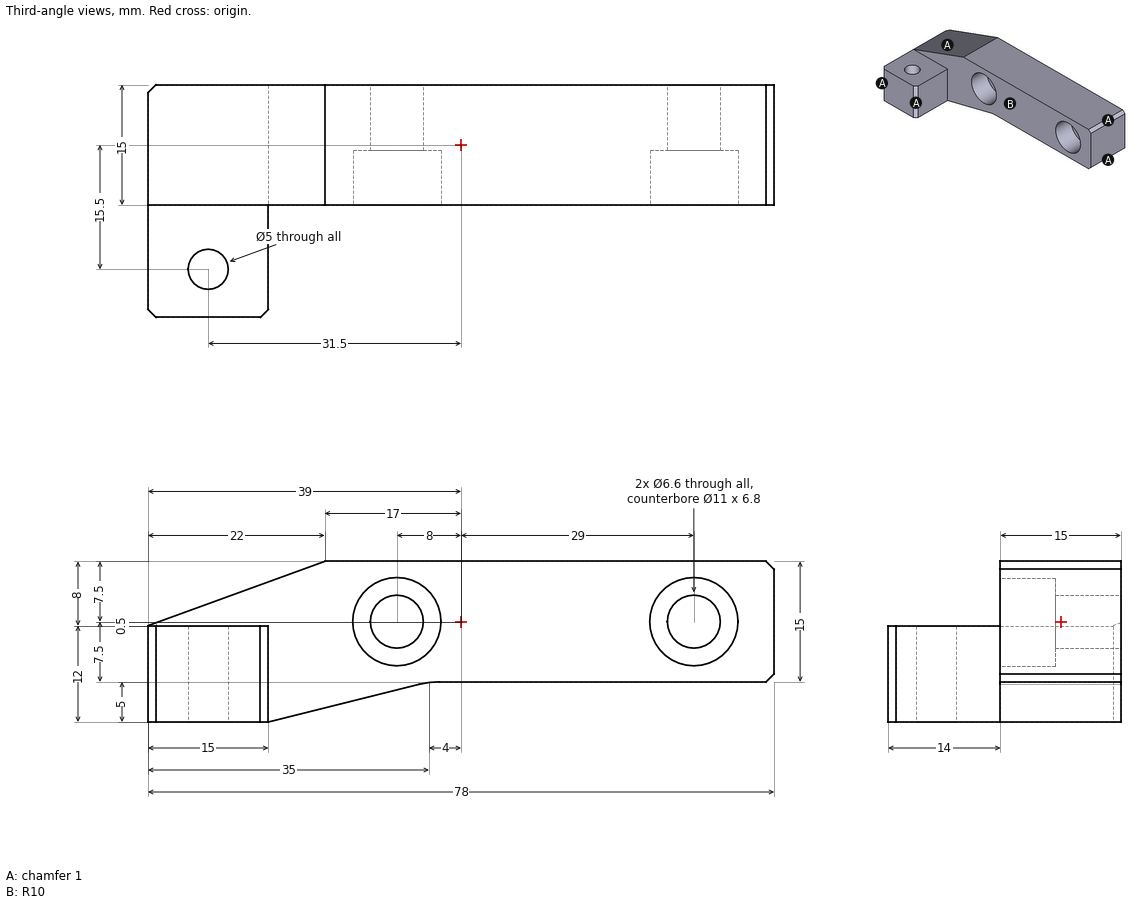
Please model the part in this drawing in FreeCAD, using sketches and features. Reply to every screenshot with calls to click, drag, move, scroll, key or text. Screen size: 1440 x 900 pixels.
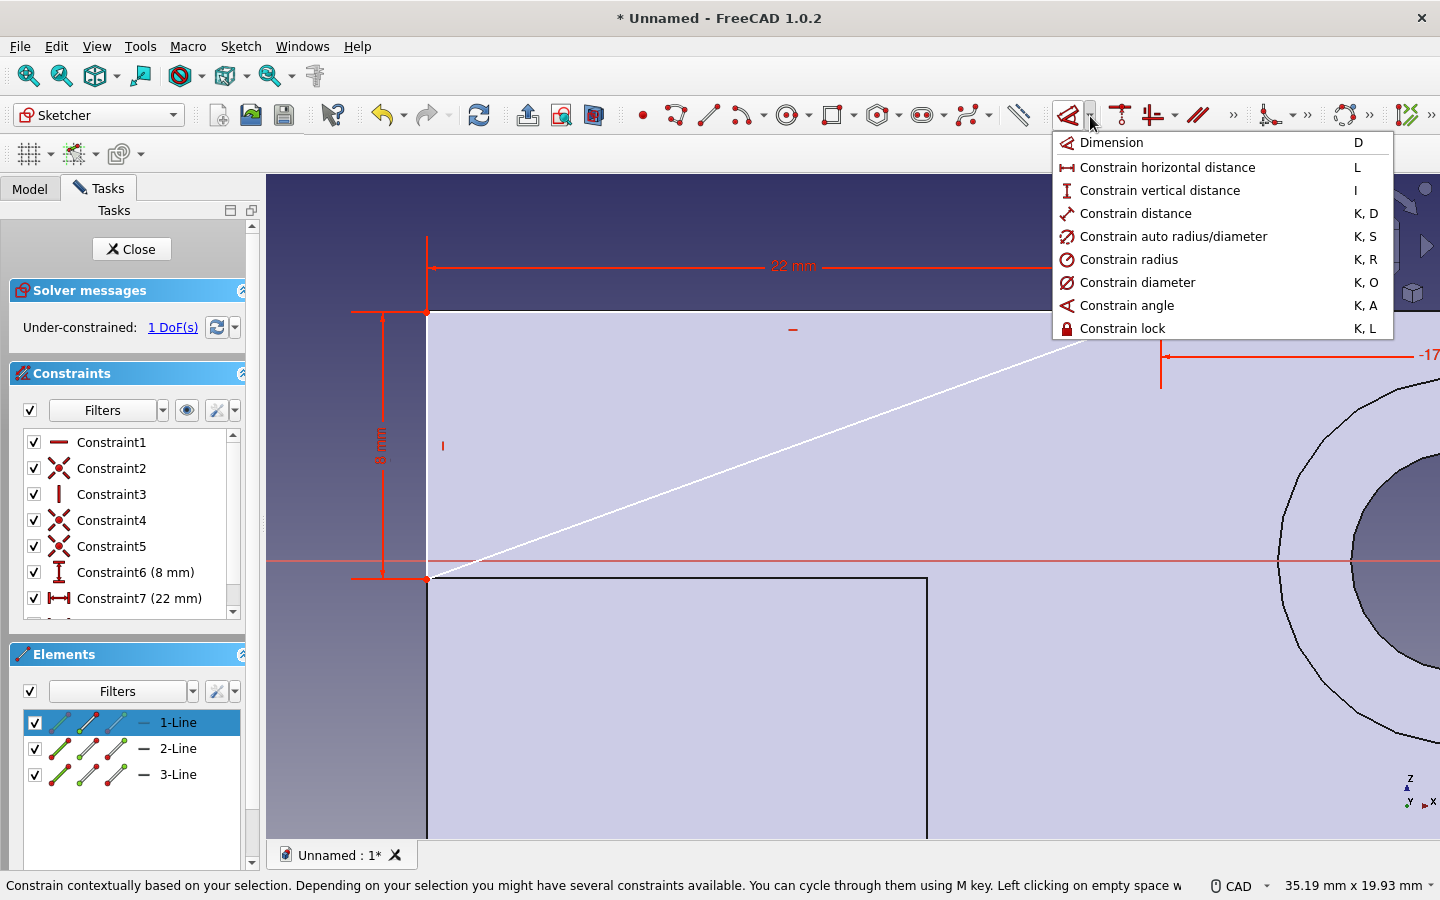
click(1223, 190)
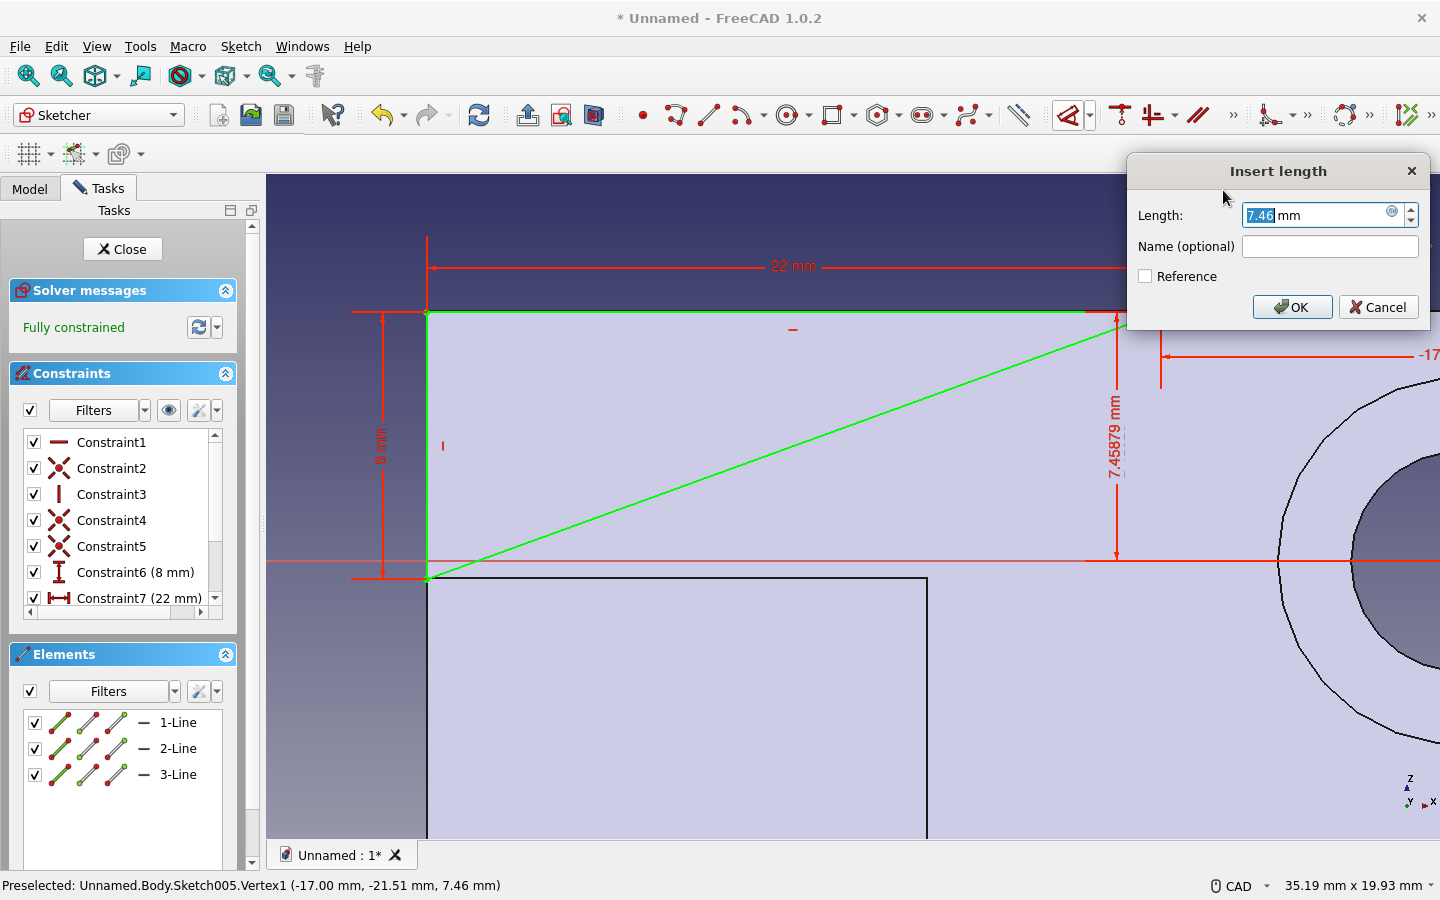
text(7.5)
key(Return)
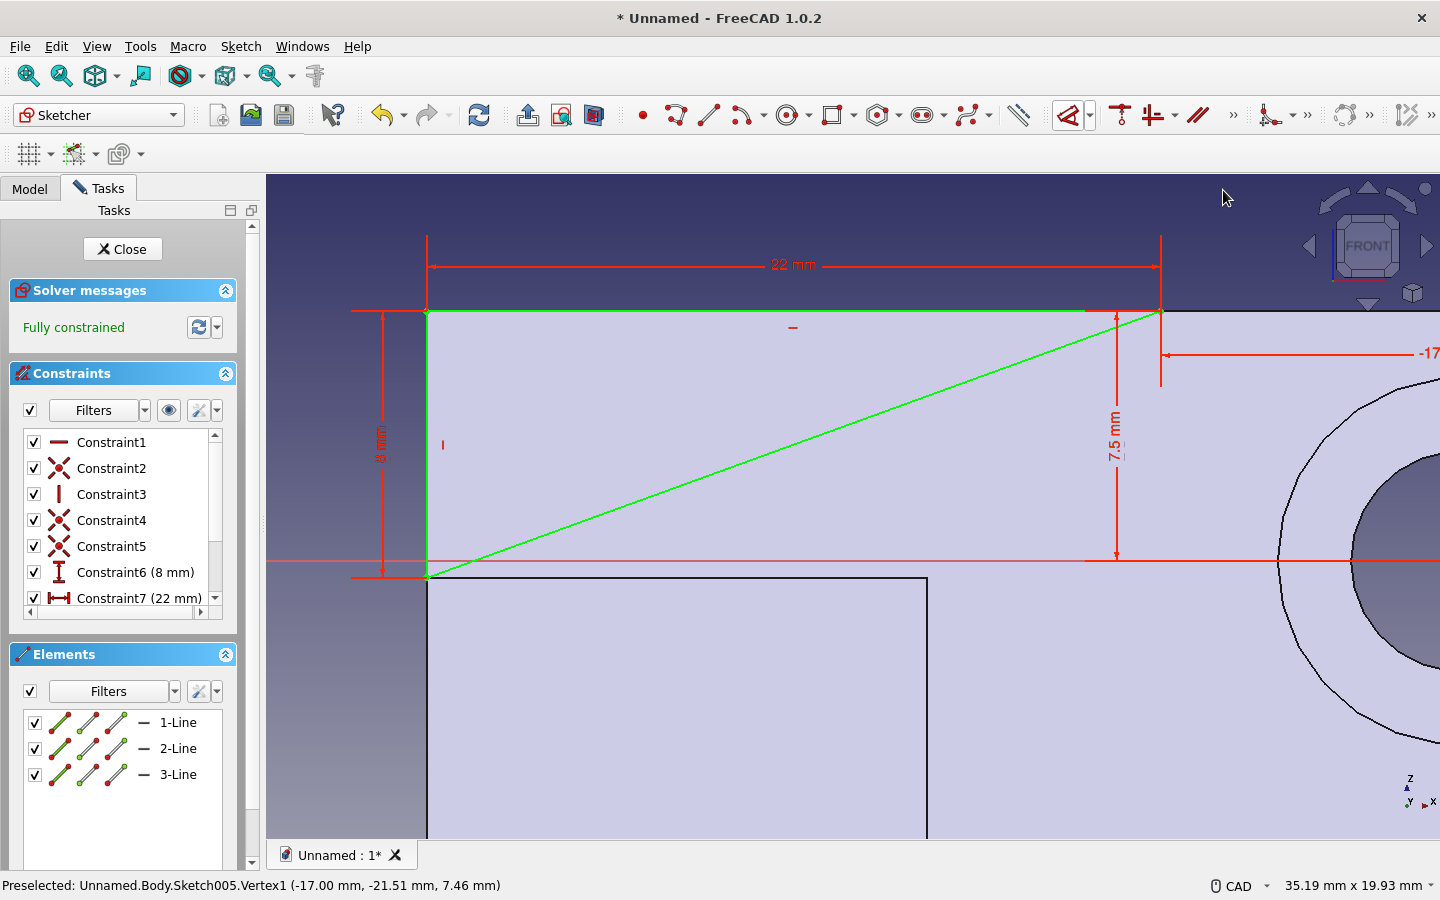
click(123, 249)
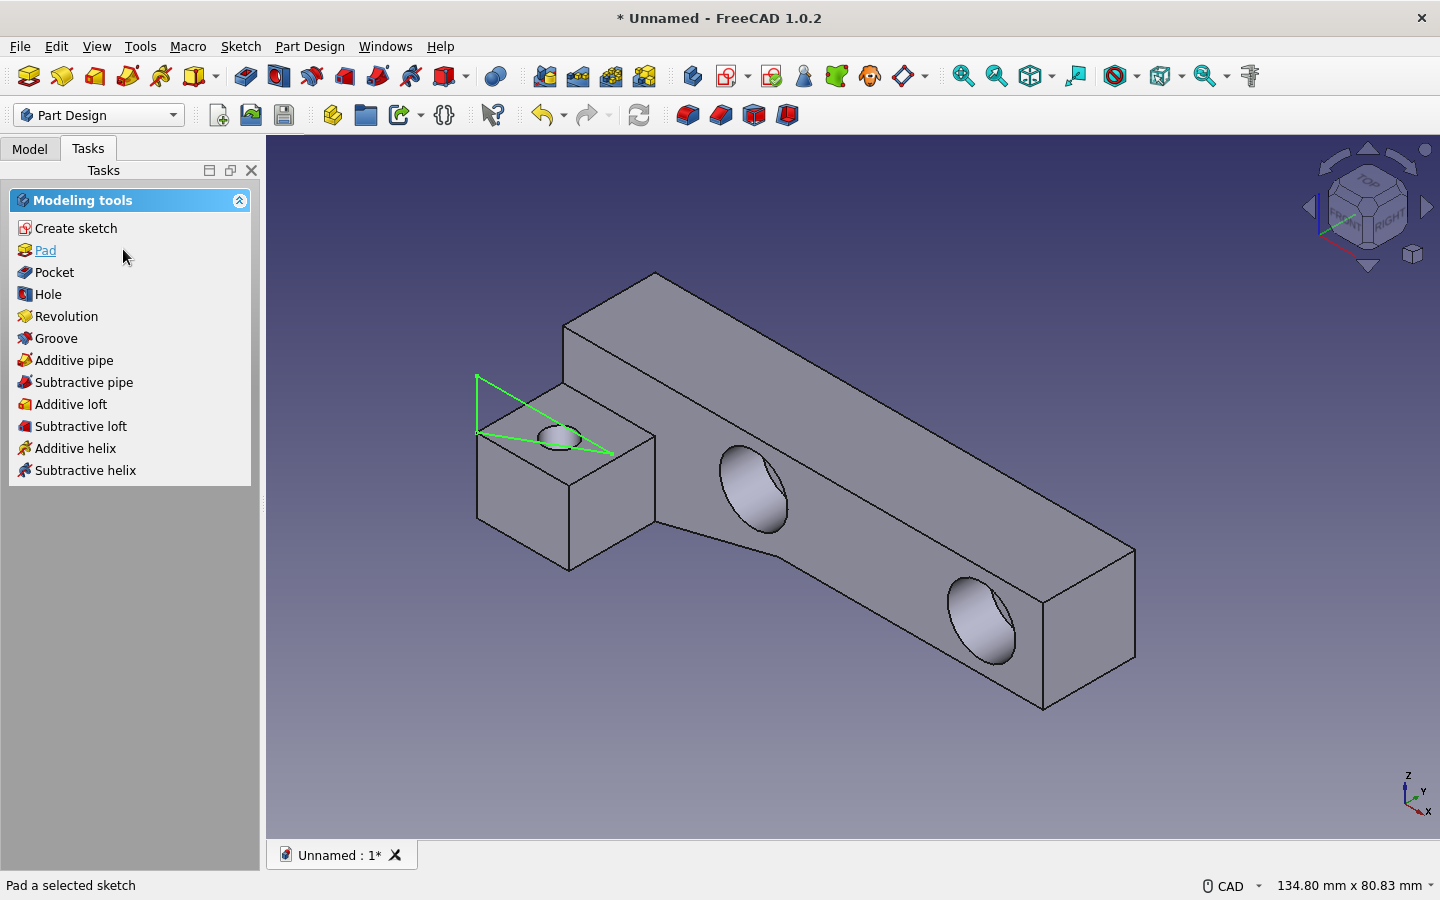
click(246, 76)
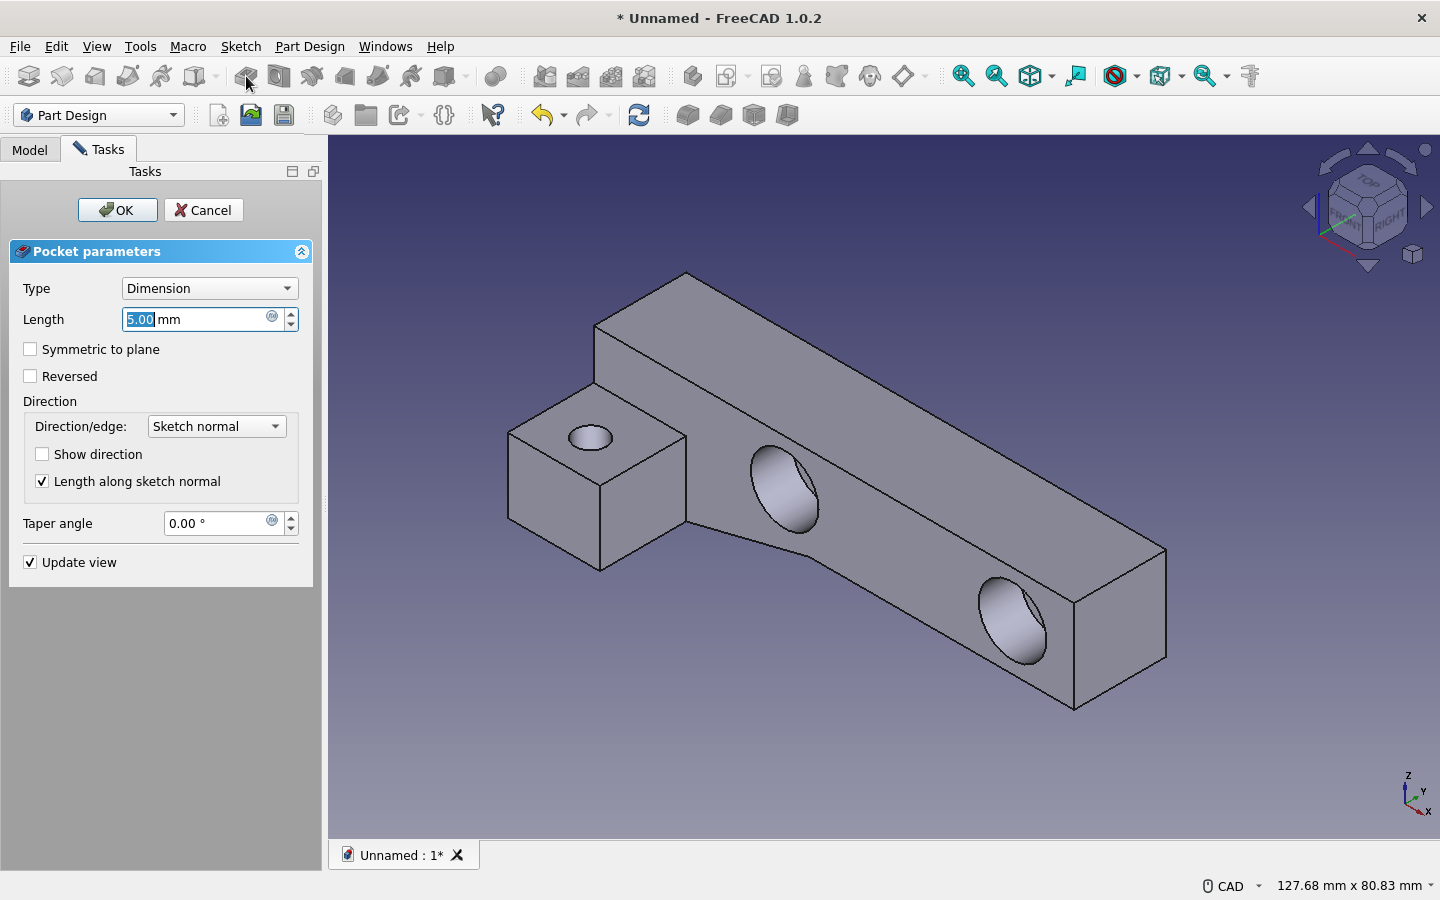
click(210, 288)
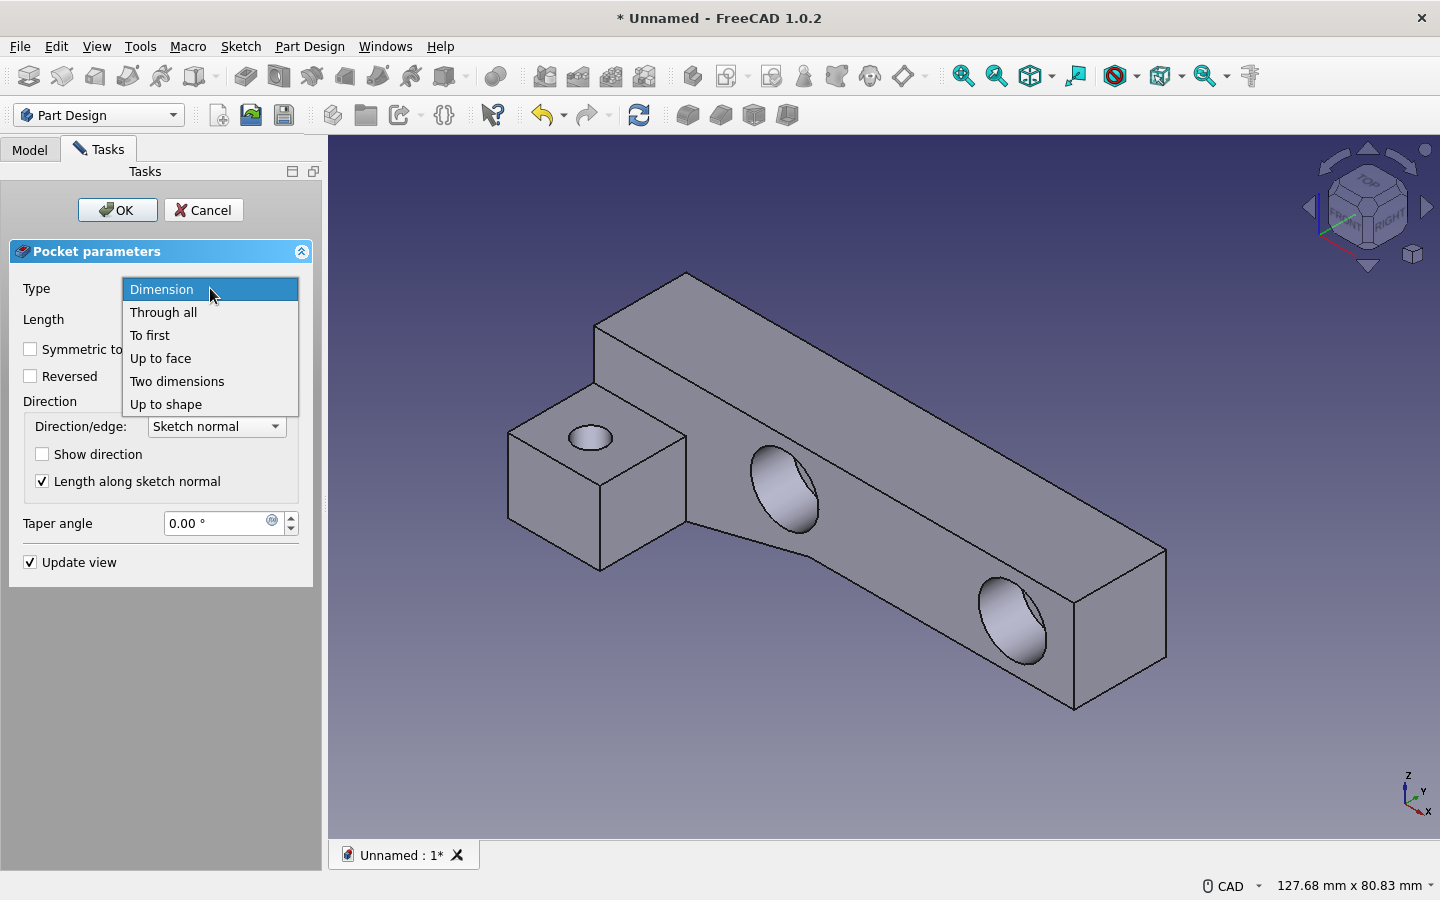
click(208, 312)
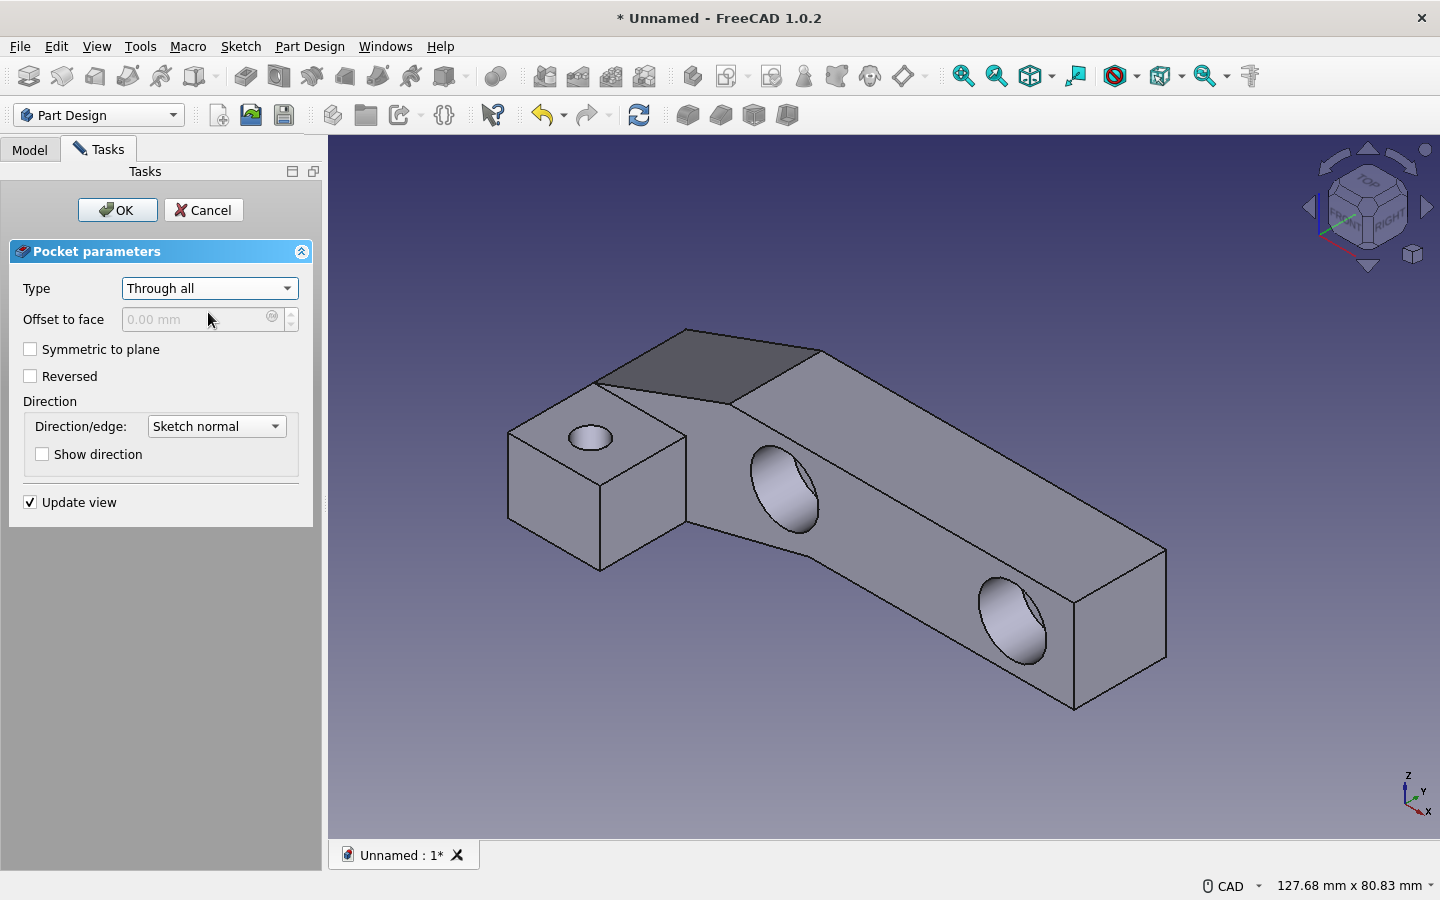
click(118, 210)